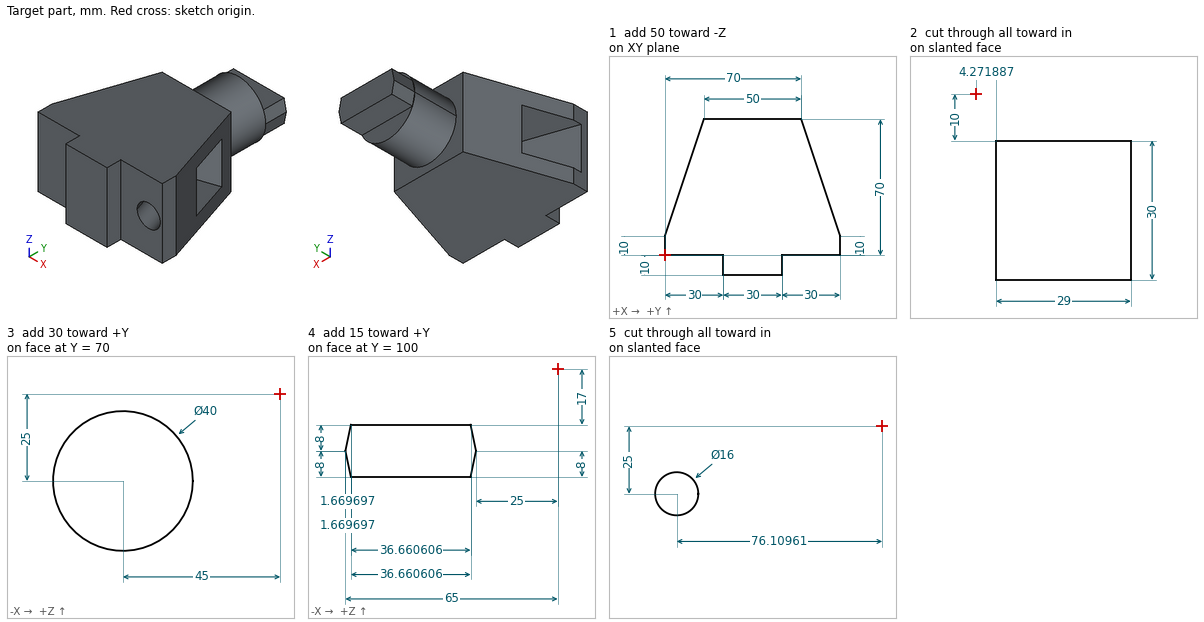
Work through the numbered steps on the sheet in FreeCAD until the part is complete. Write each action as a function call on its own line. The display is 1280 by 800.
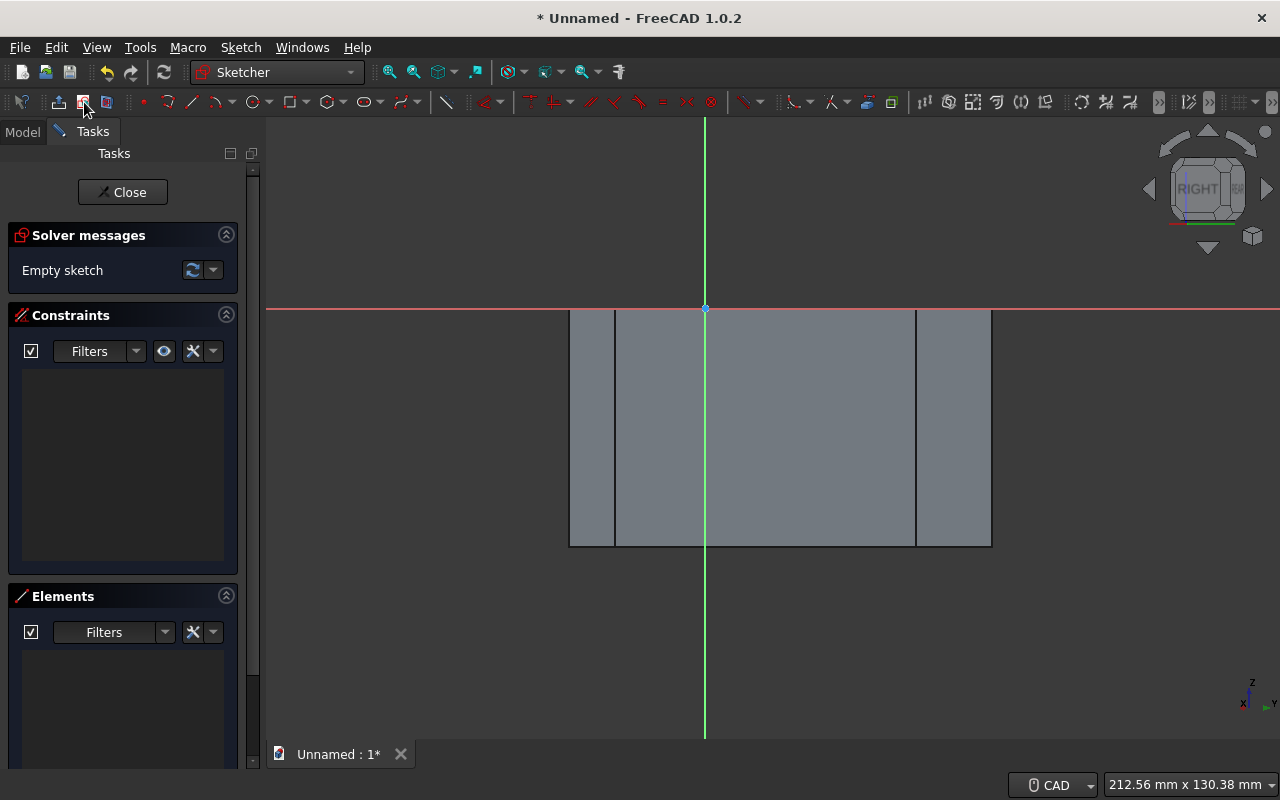
scroll(850, 385, up, 4)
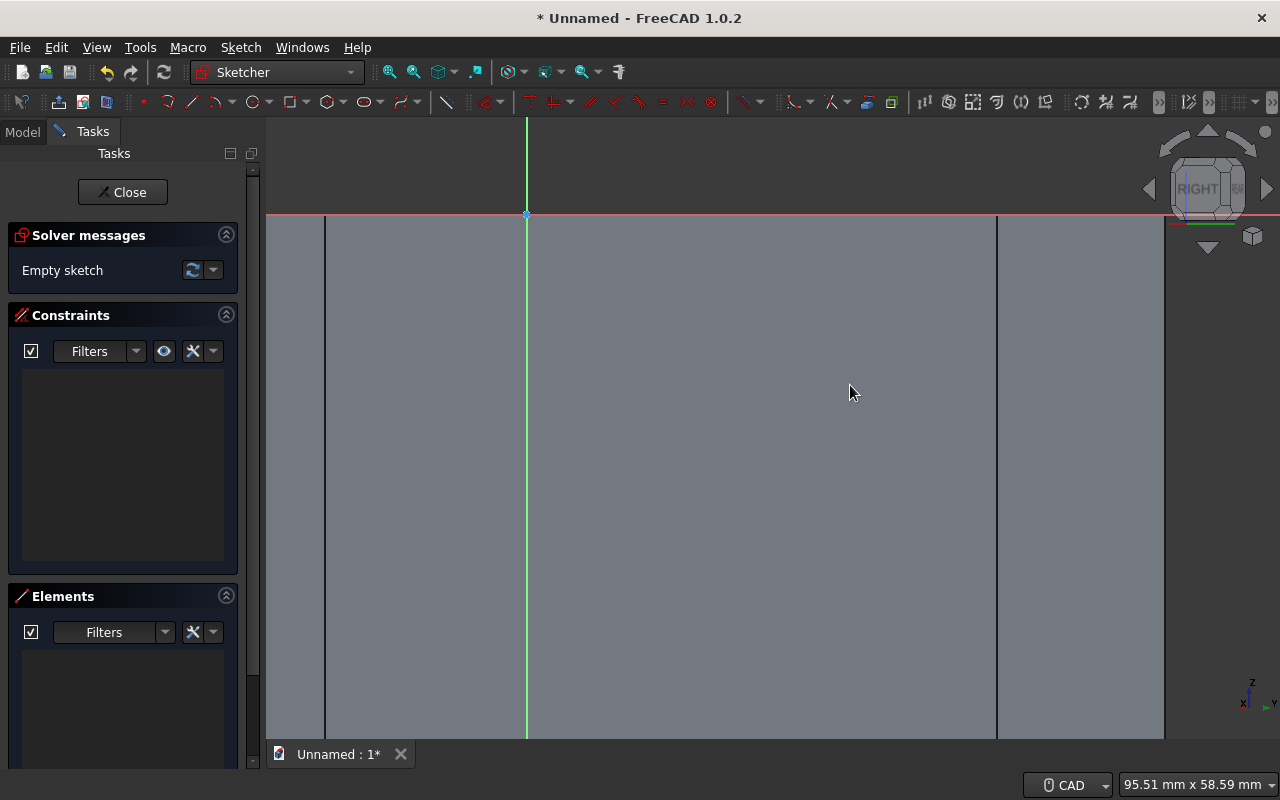
key(g)
key(r)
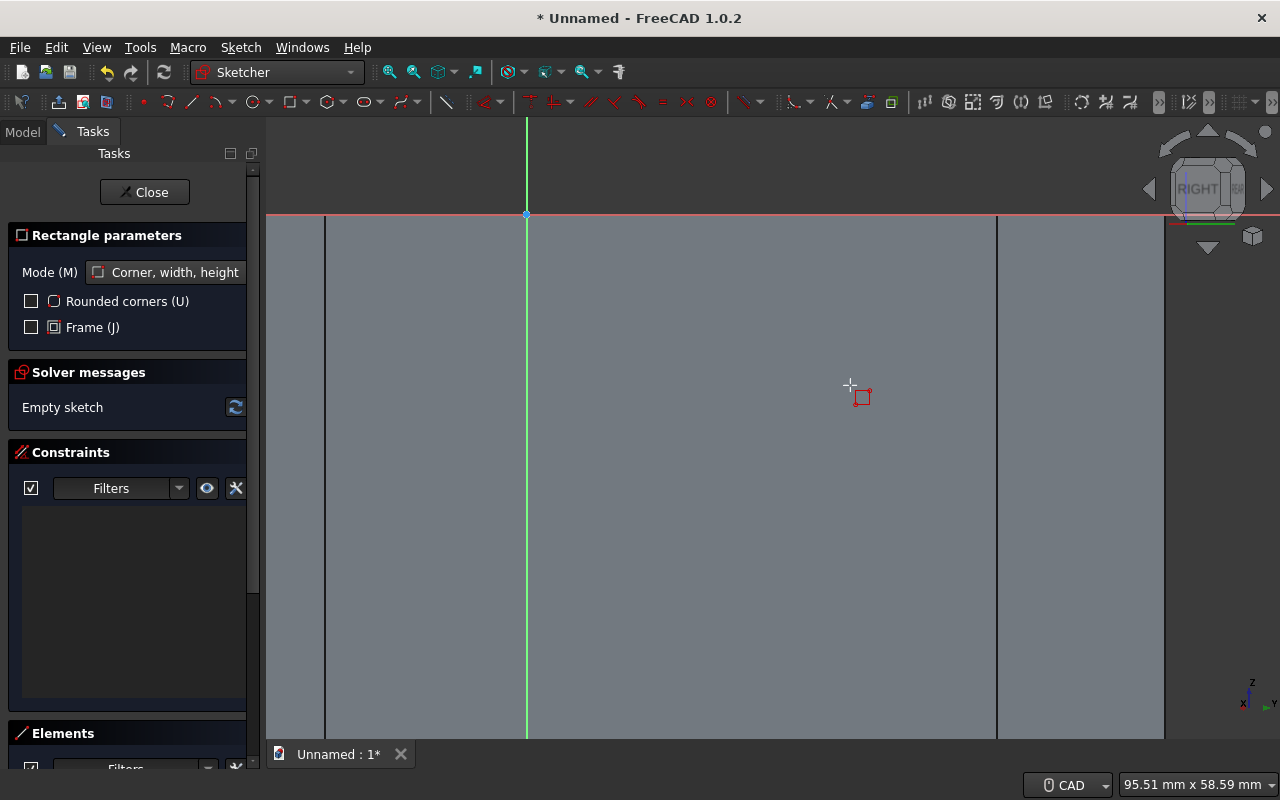
click(572, 321)
move(880, 639)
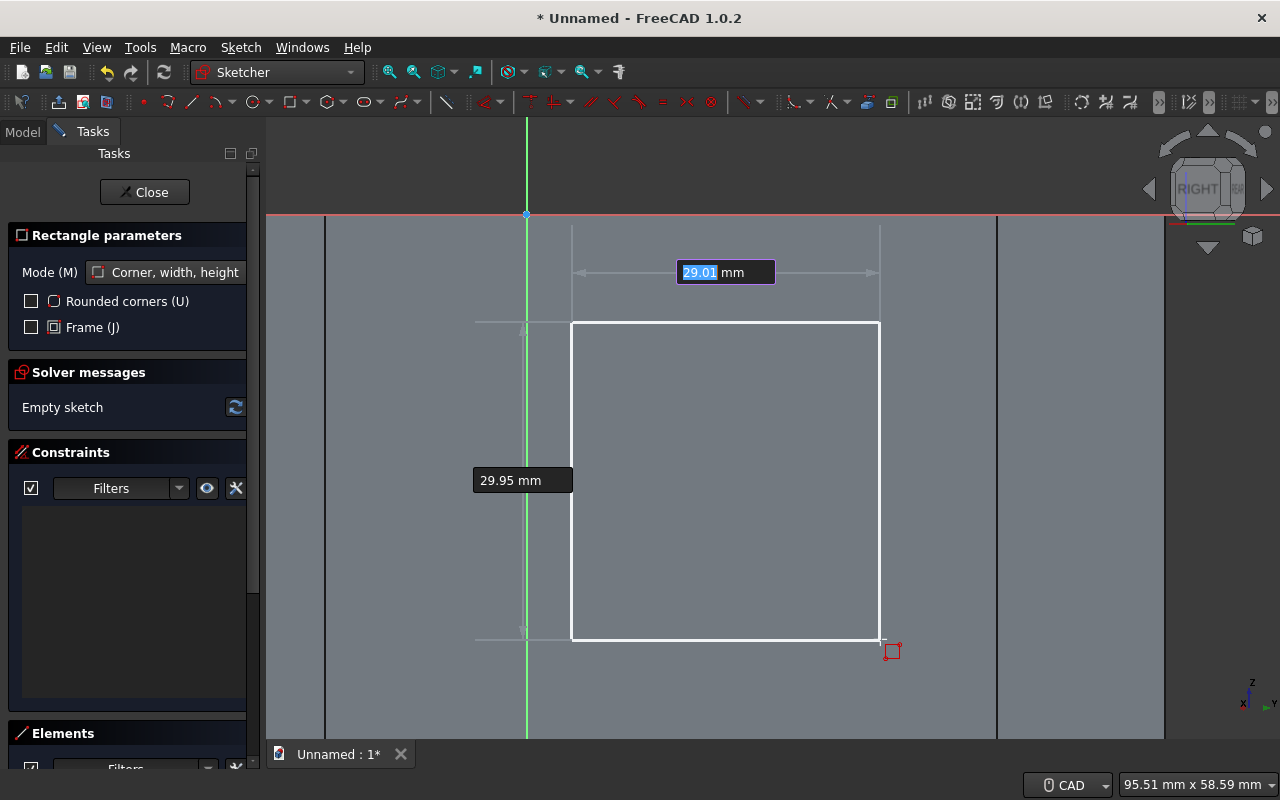
text(29)
key(Tab)
text(30)
key(Return)
key(Escape)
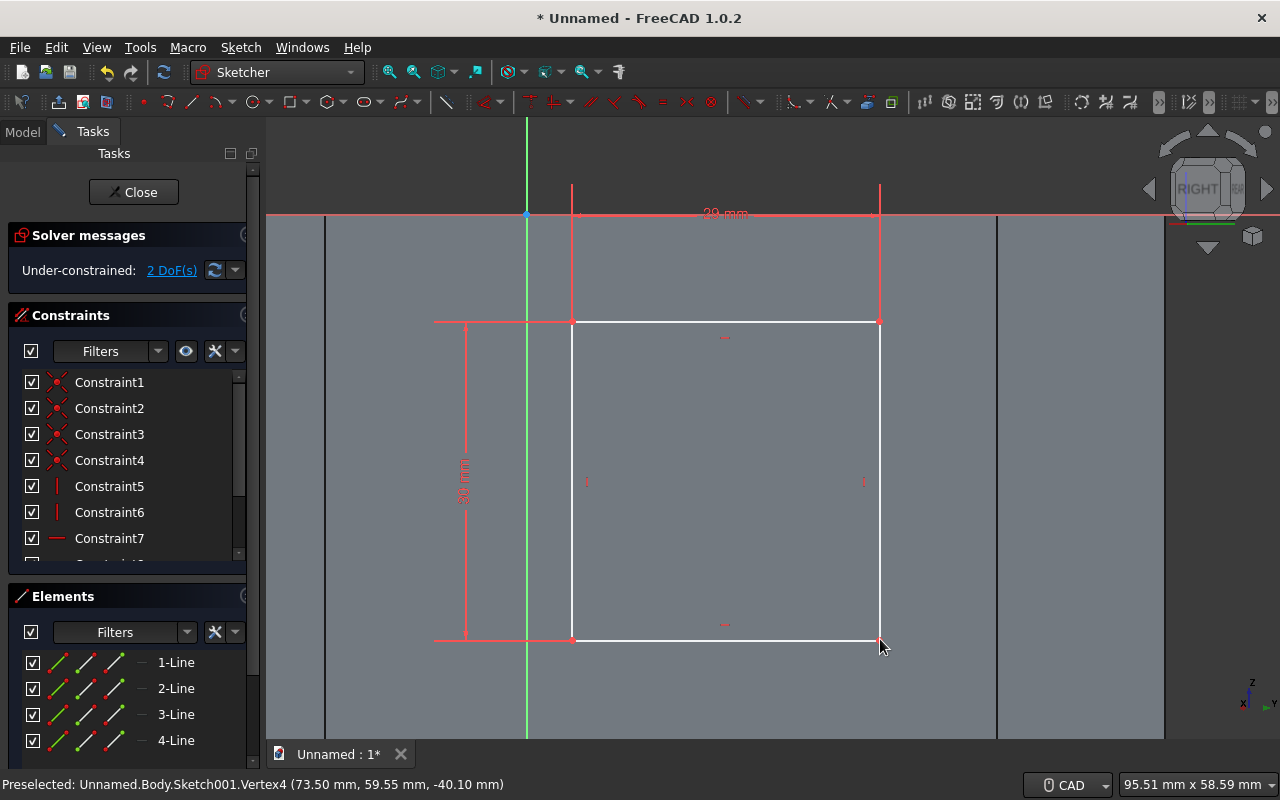
key(d)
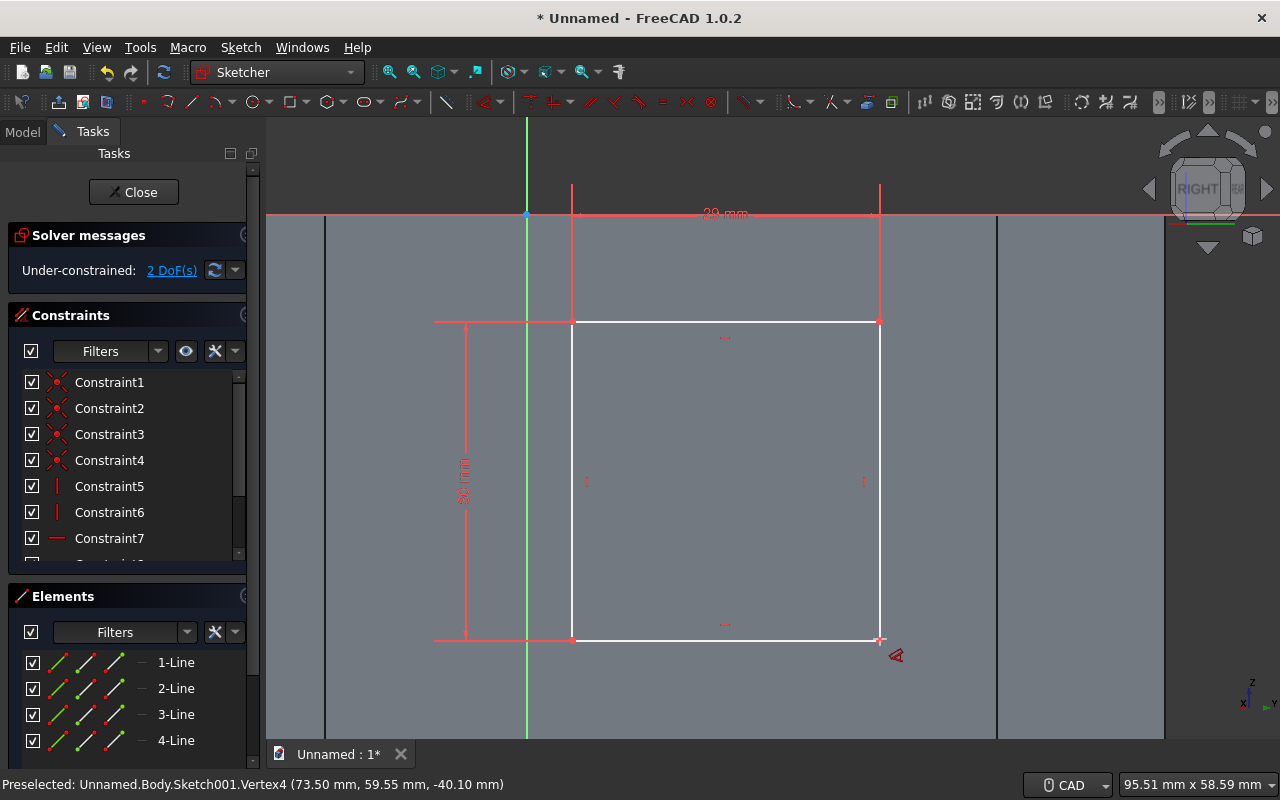
click(572, 322)
click(493, 268)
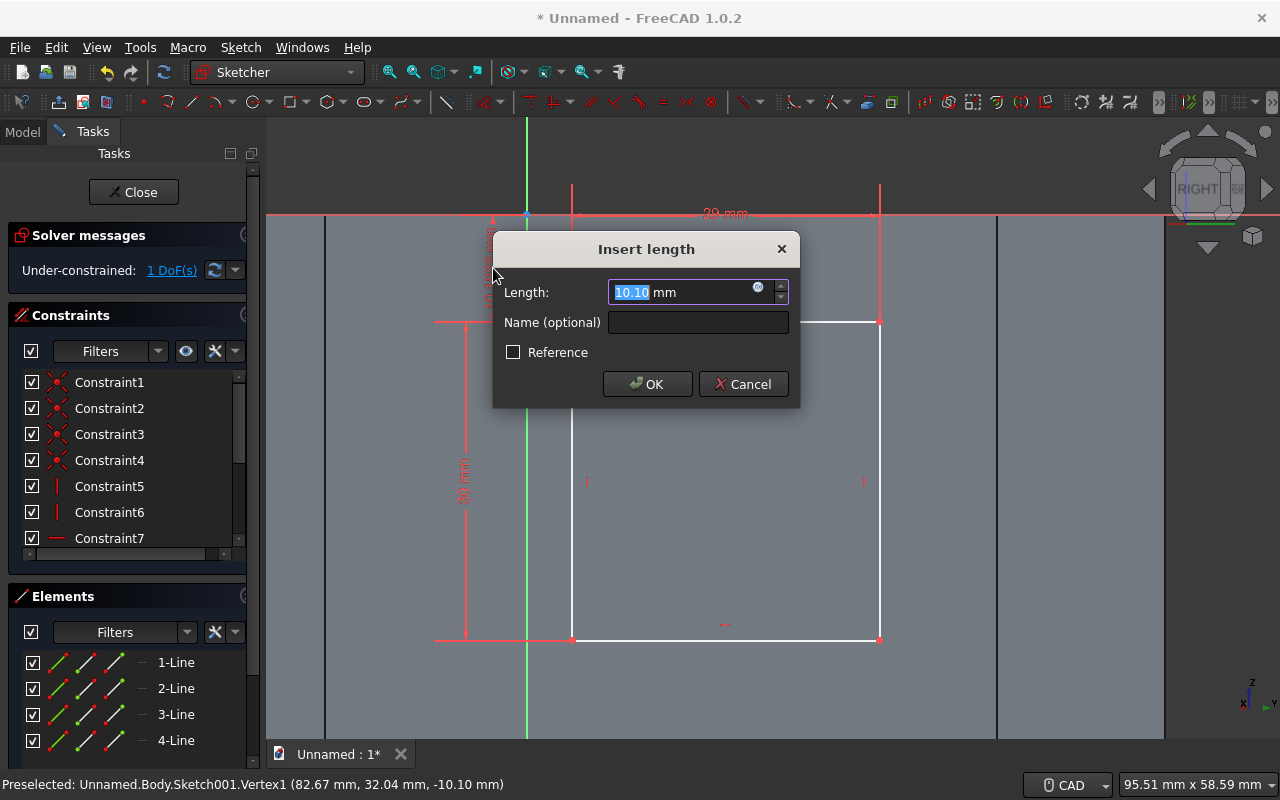
text(10)
key(Return)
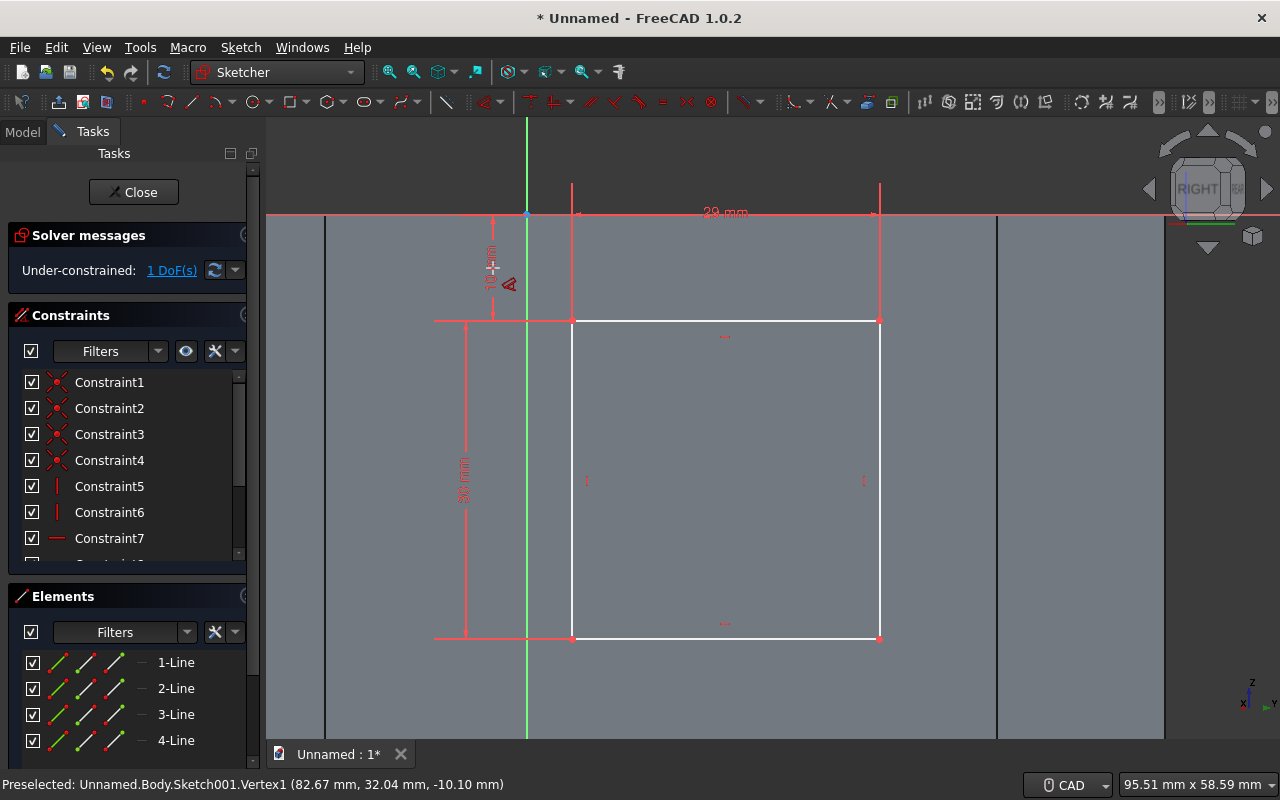
click(572, 321)
click(549, 181)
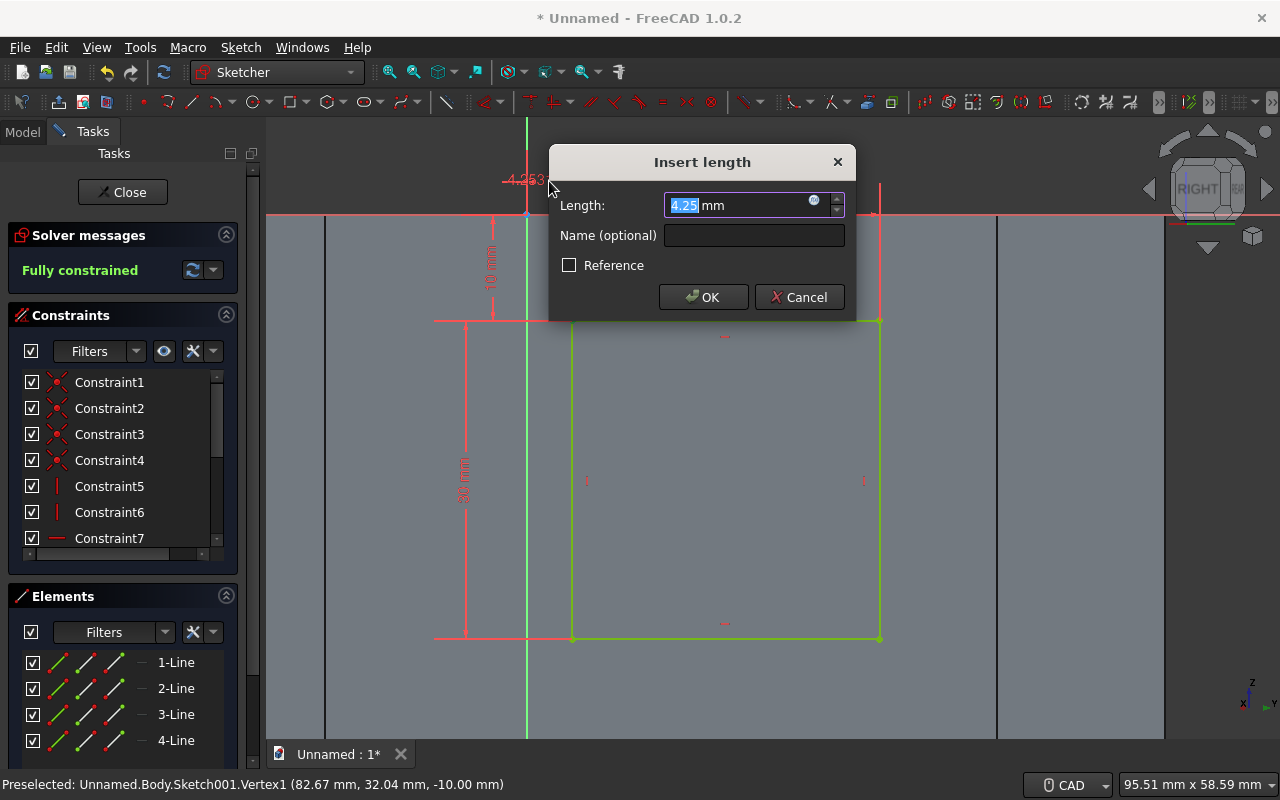
text(4.271887)
key(Return)
key(Escape)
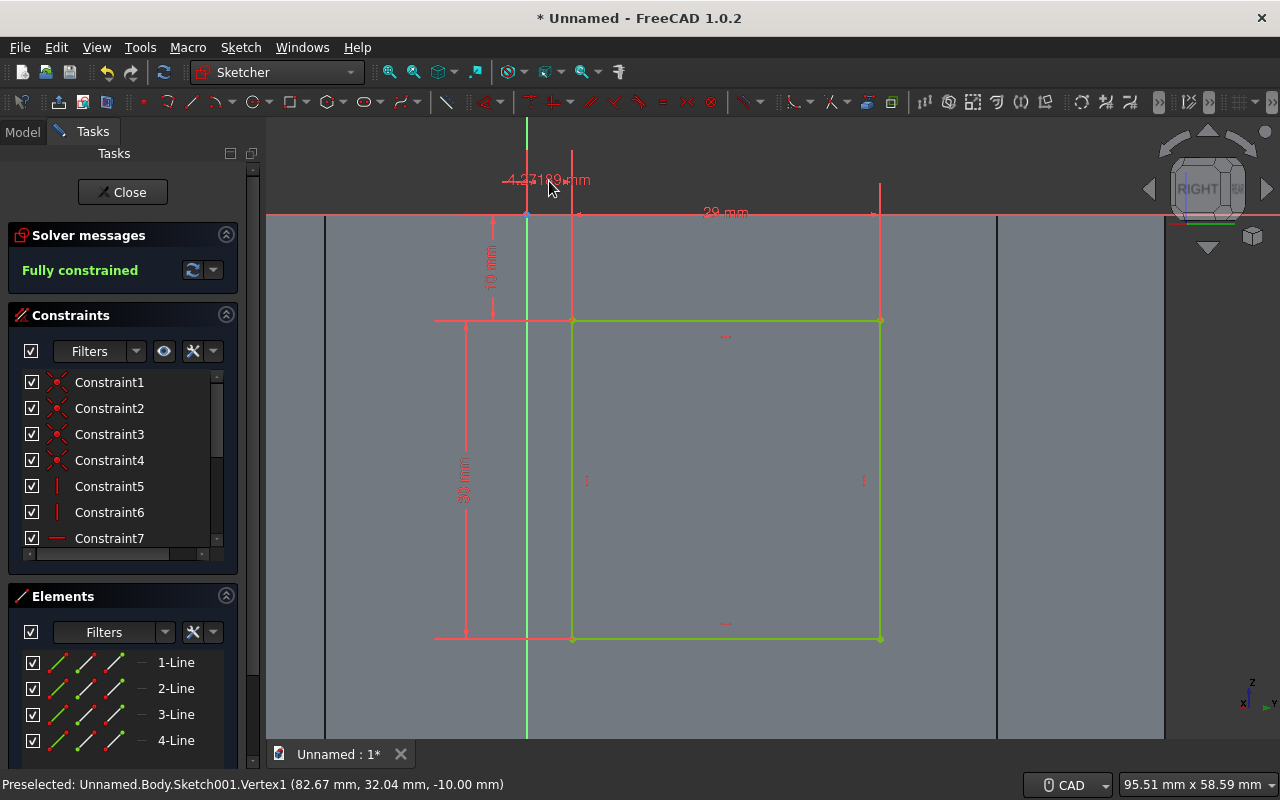
click(123, 192)